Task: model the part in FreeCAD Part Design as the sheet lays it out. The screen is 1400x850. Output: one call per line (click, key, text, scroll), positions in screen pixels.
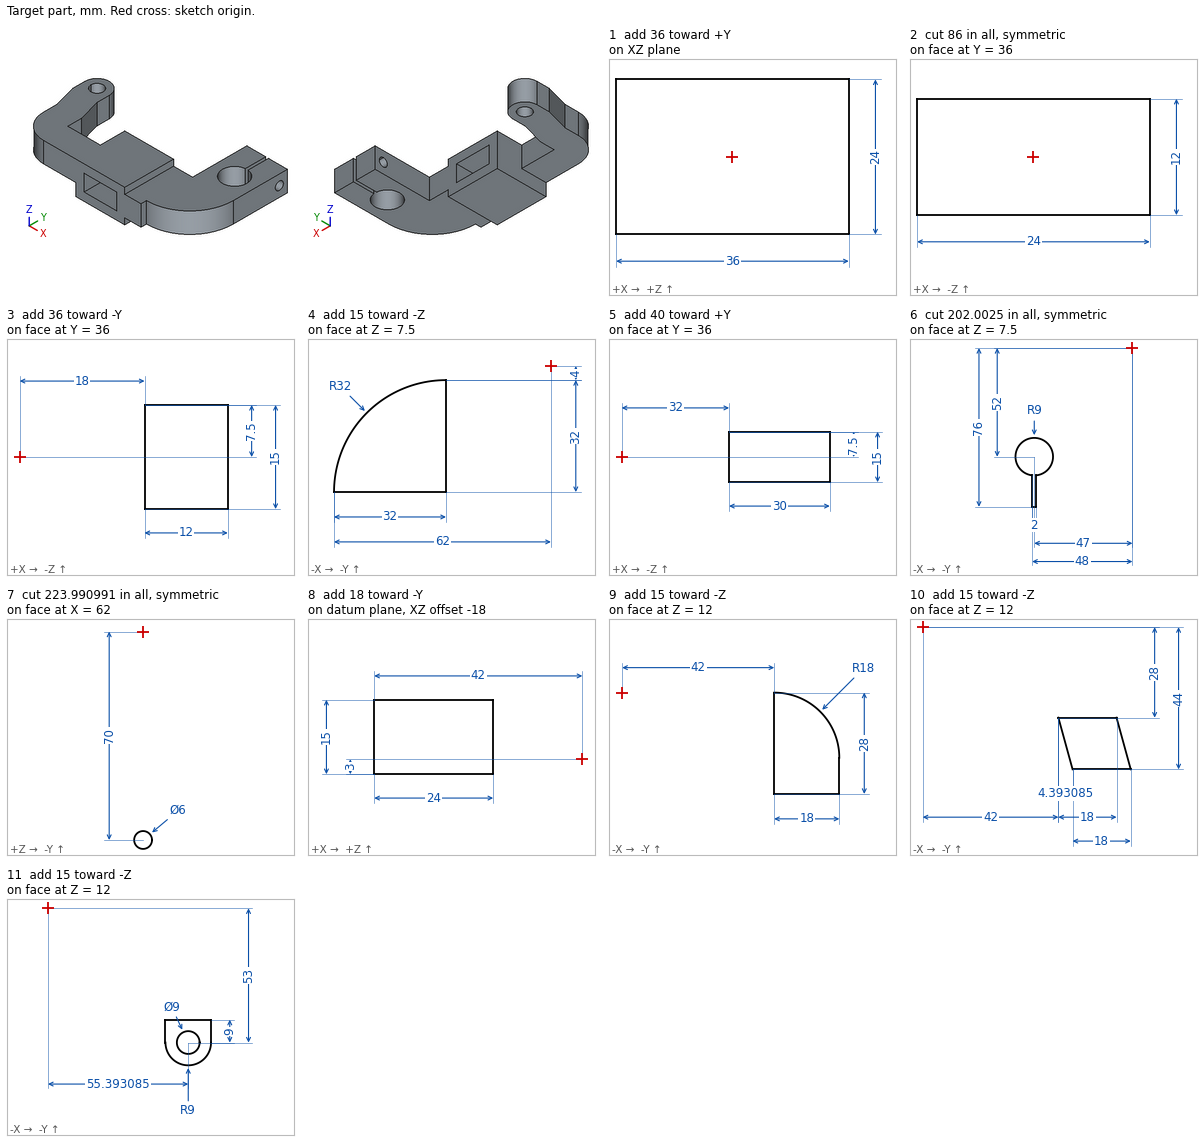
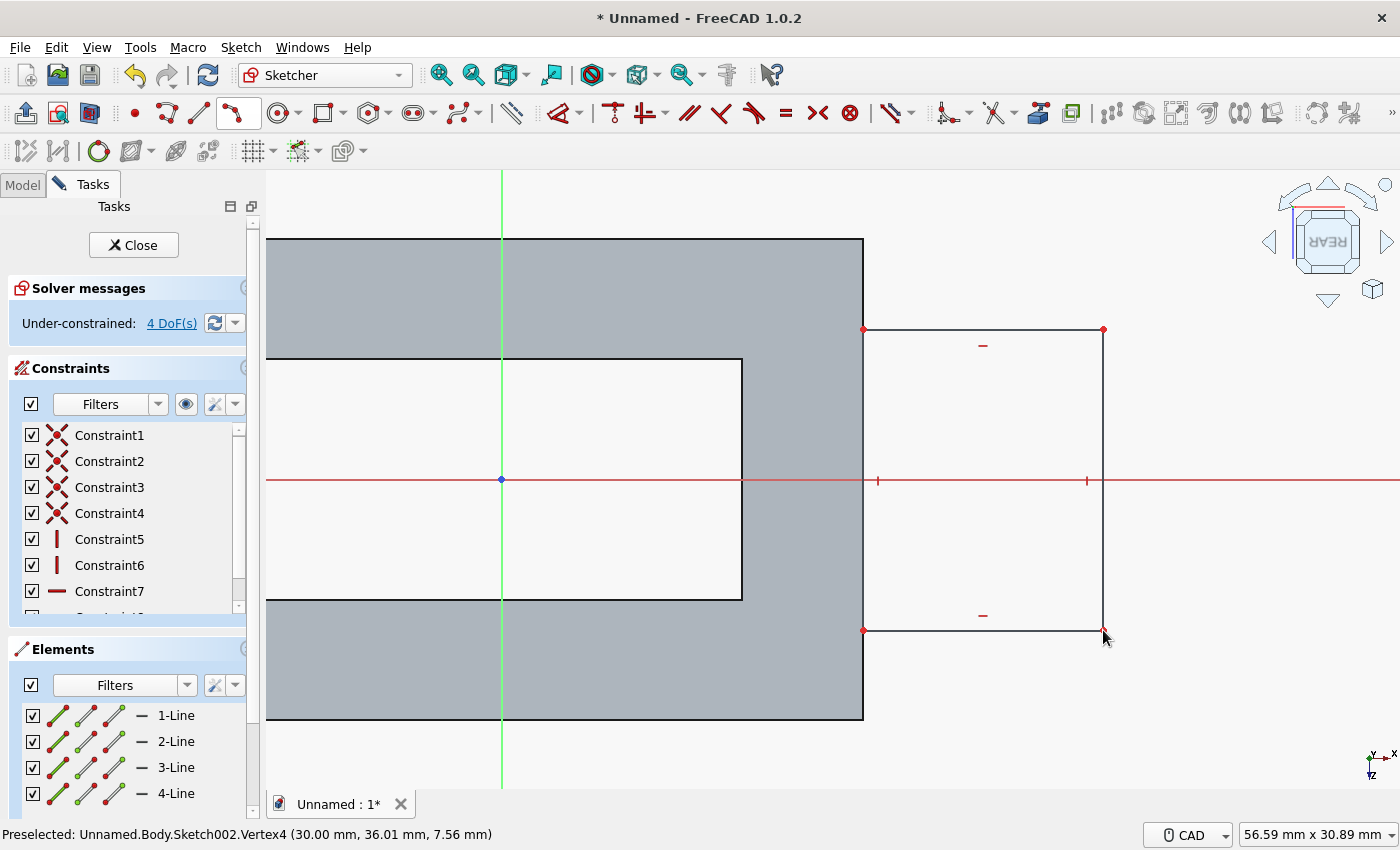
key(d)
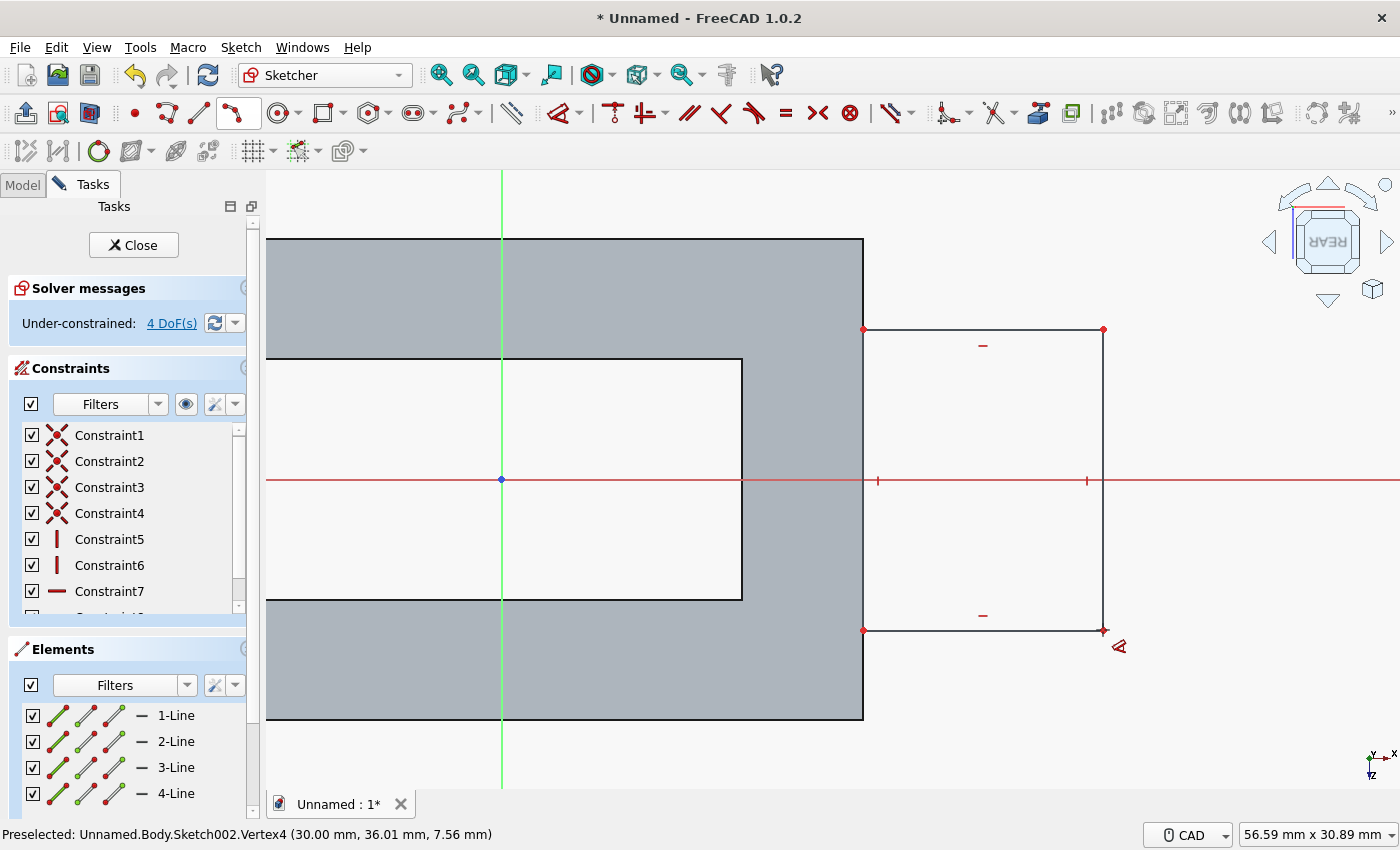
click(863, 420)
click(897, 411)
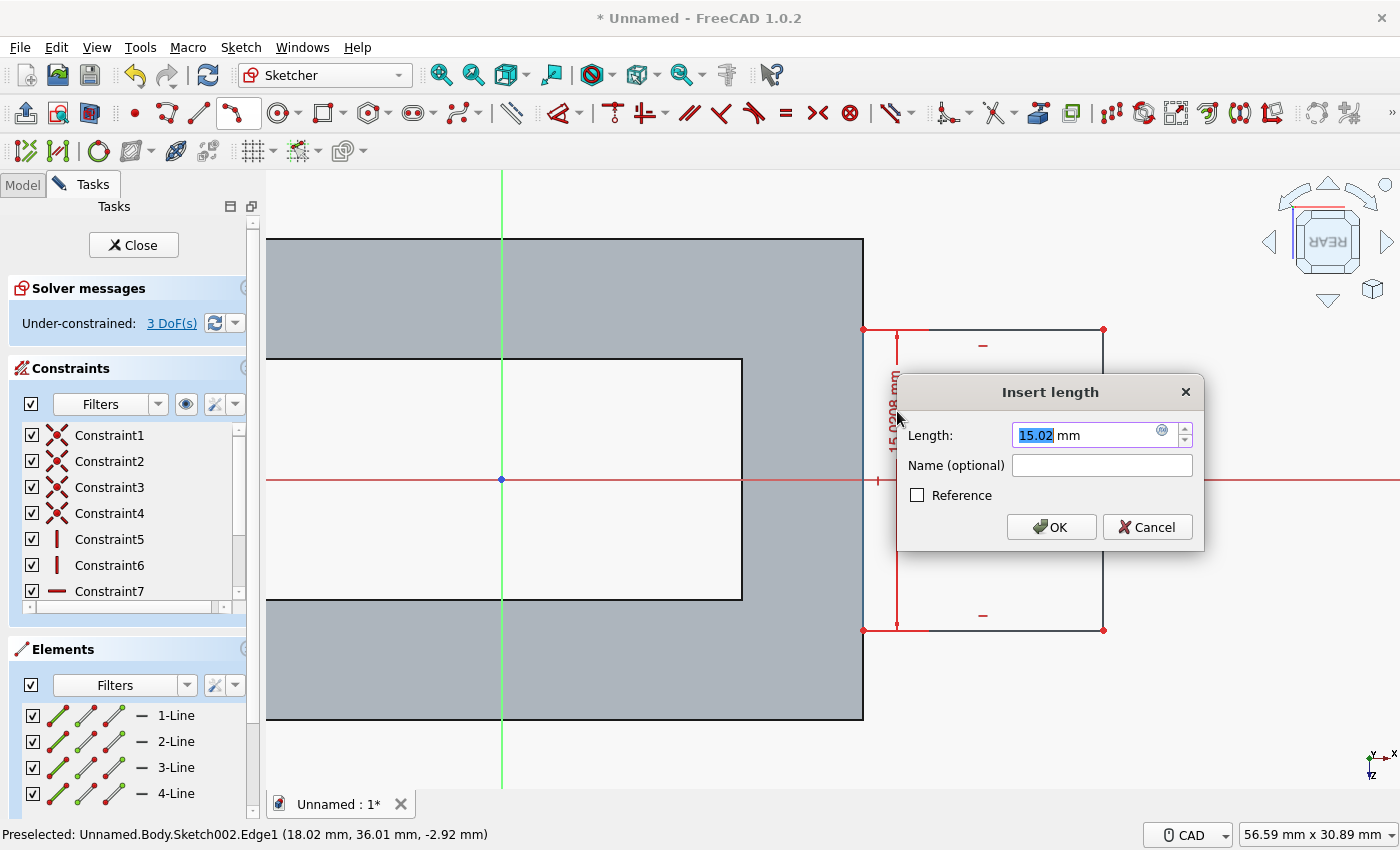
text(15)
key(Return)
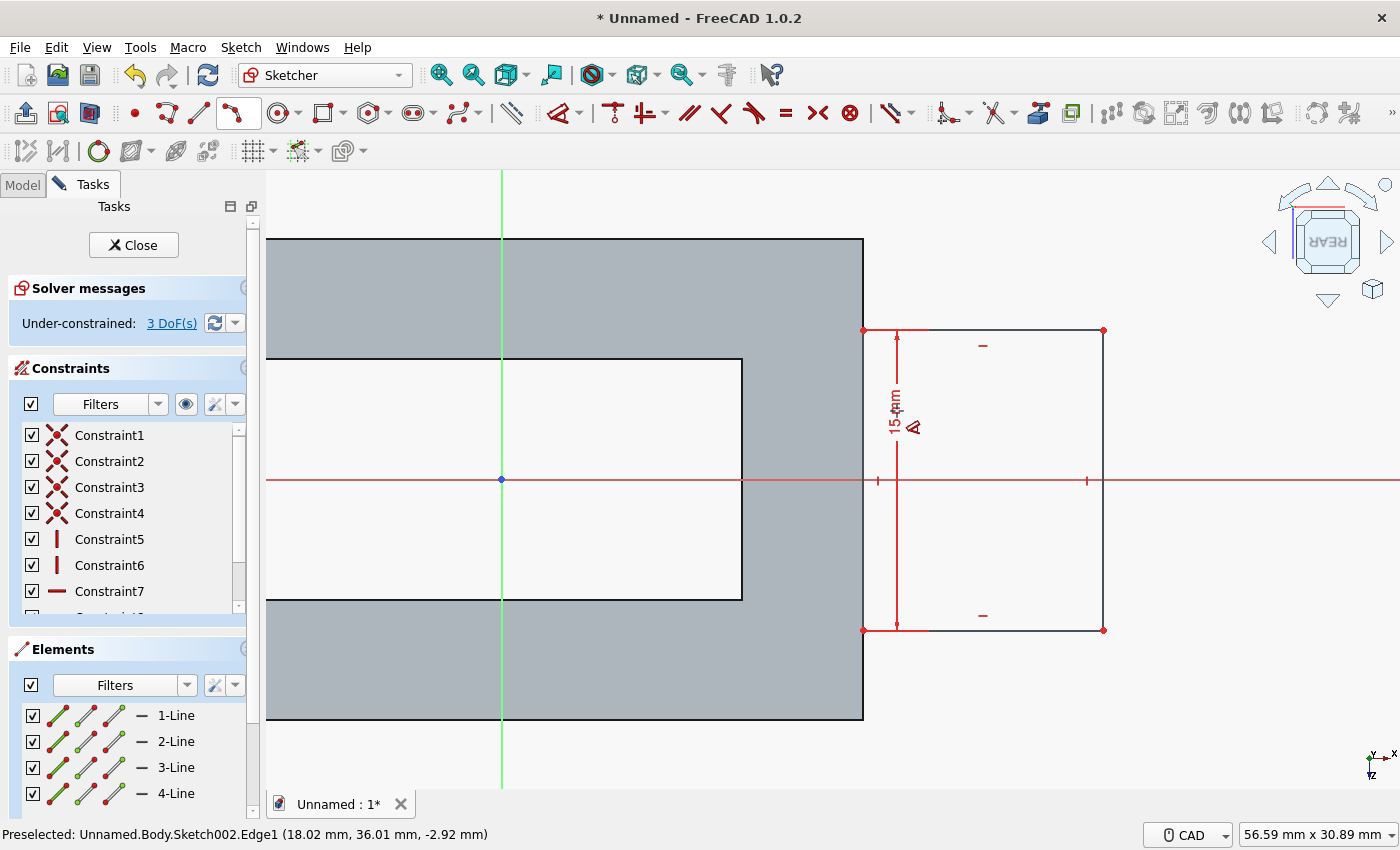
click(935, 631)
click(983, 665)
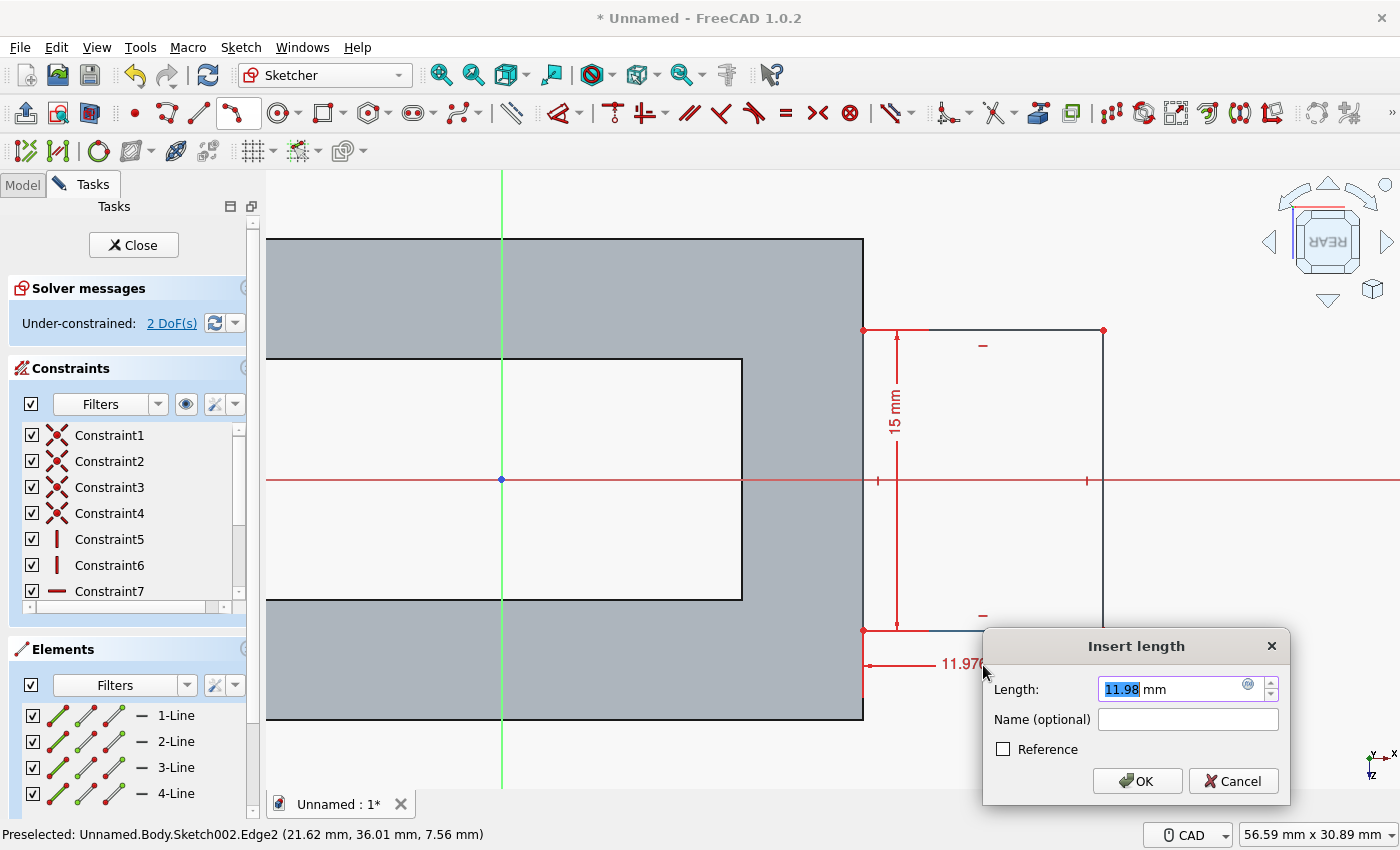
text(12)
key(Return)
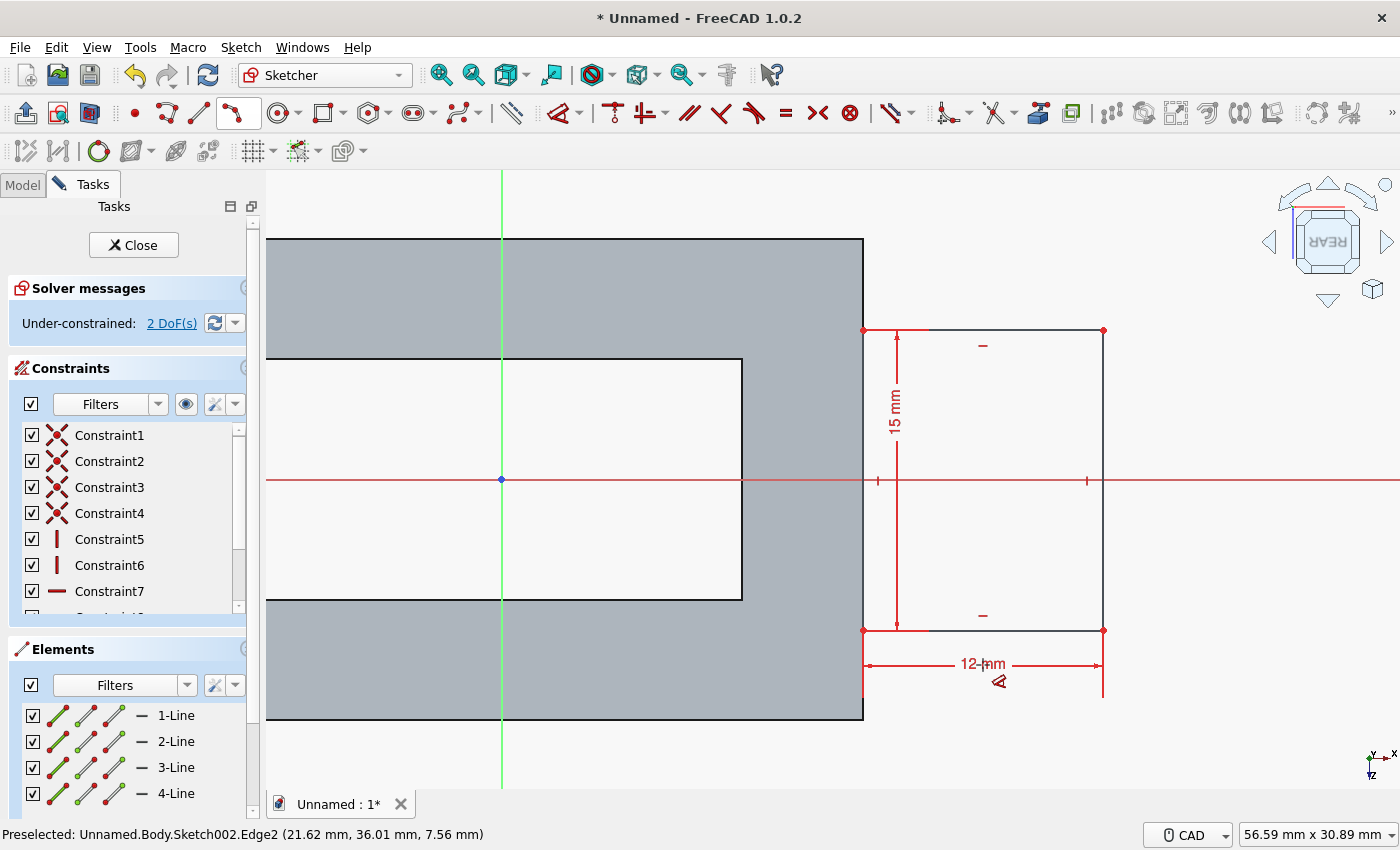
click(863, 330)
click(682, 296)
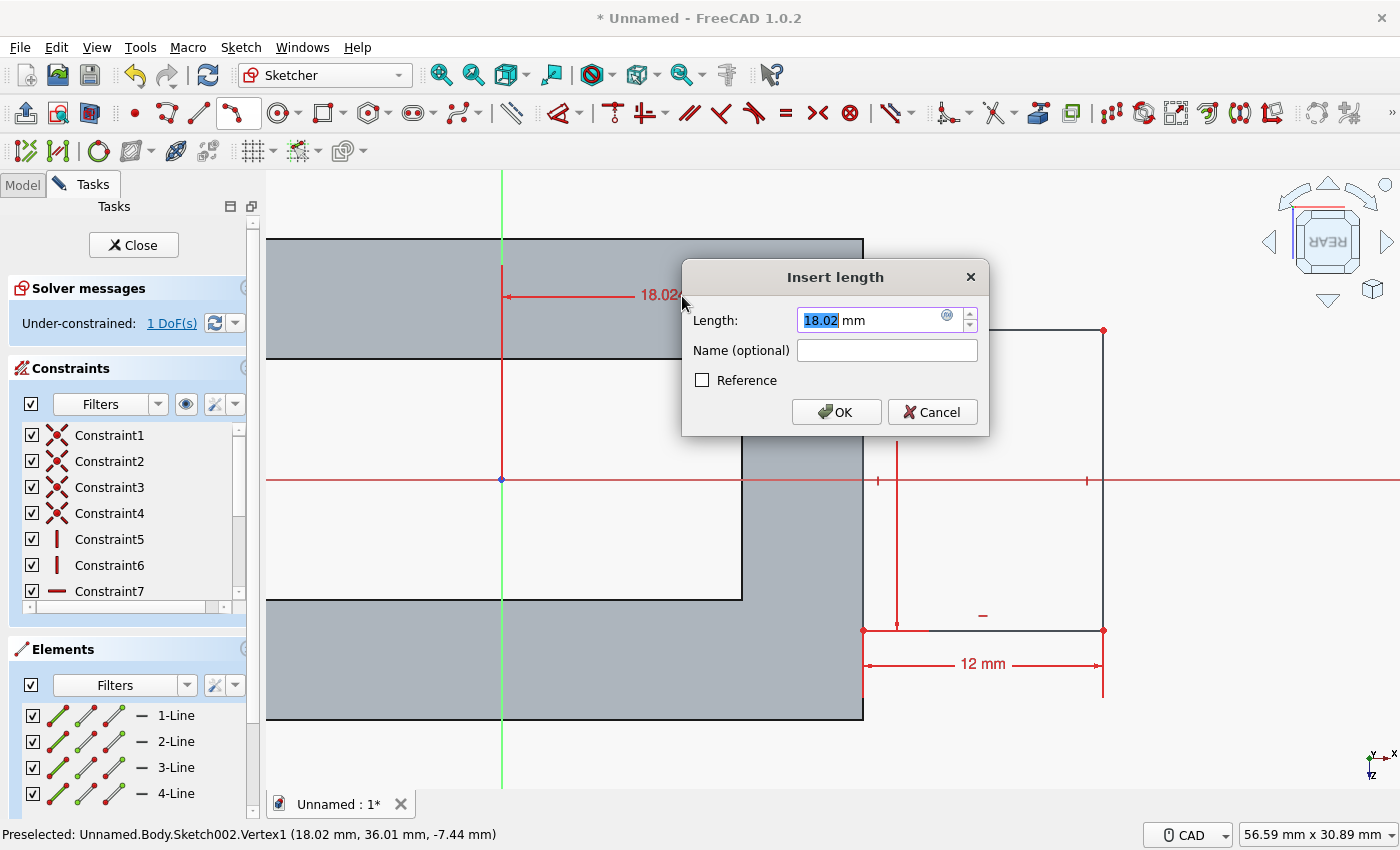
text(18)
key(Return)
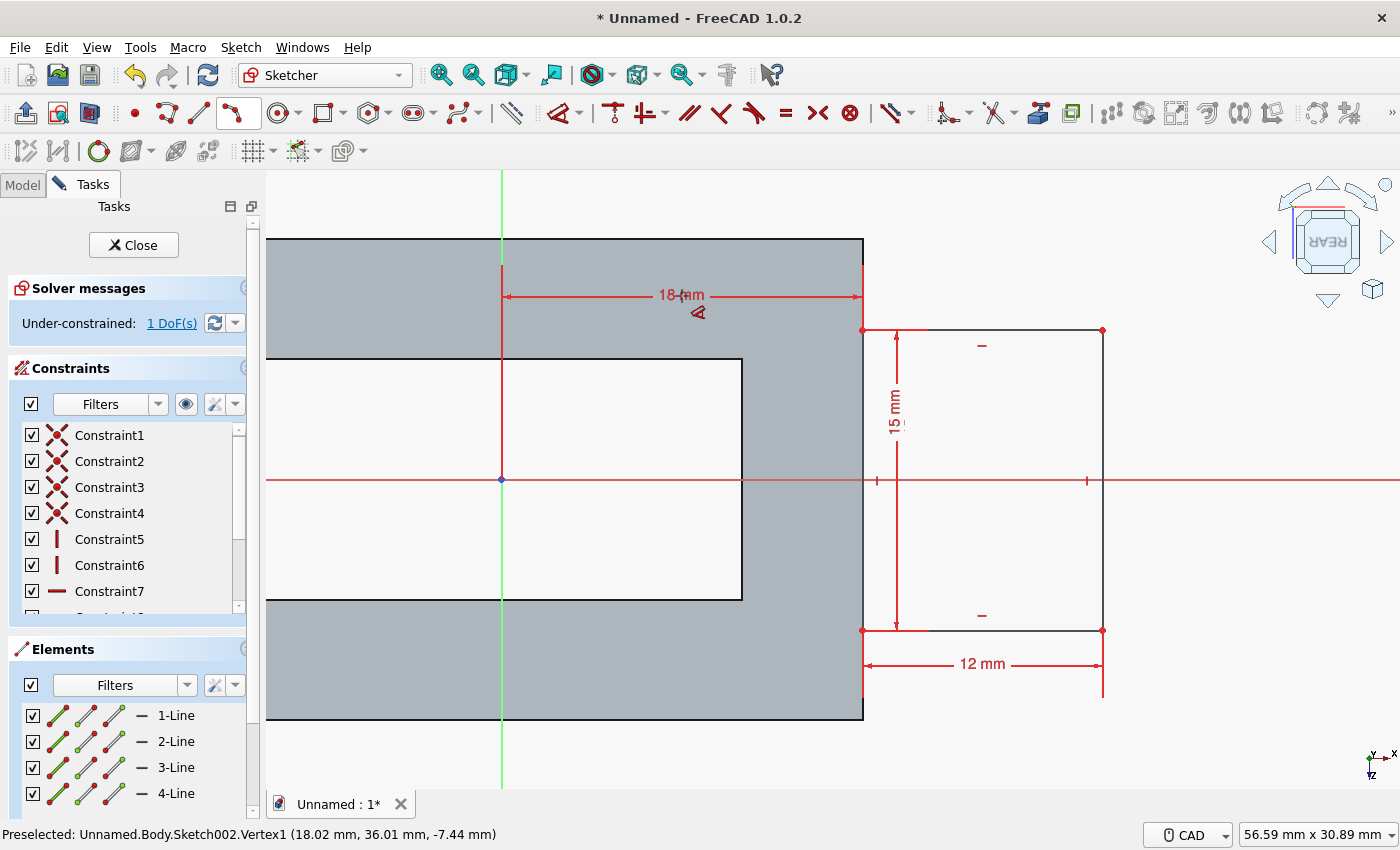
click(863, 330)
click(468, 405)